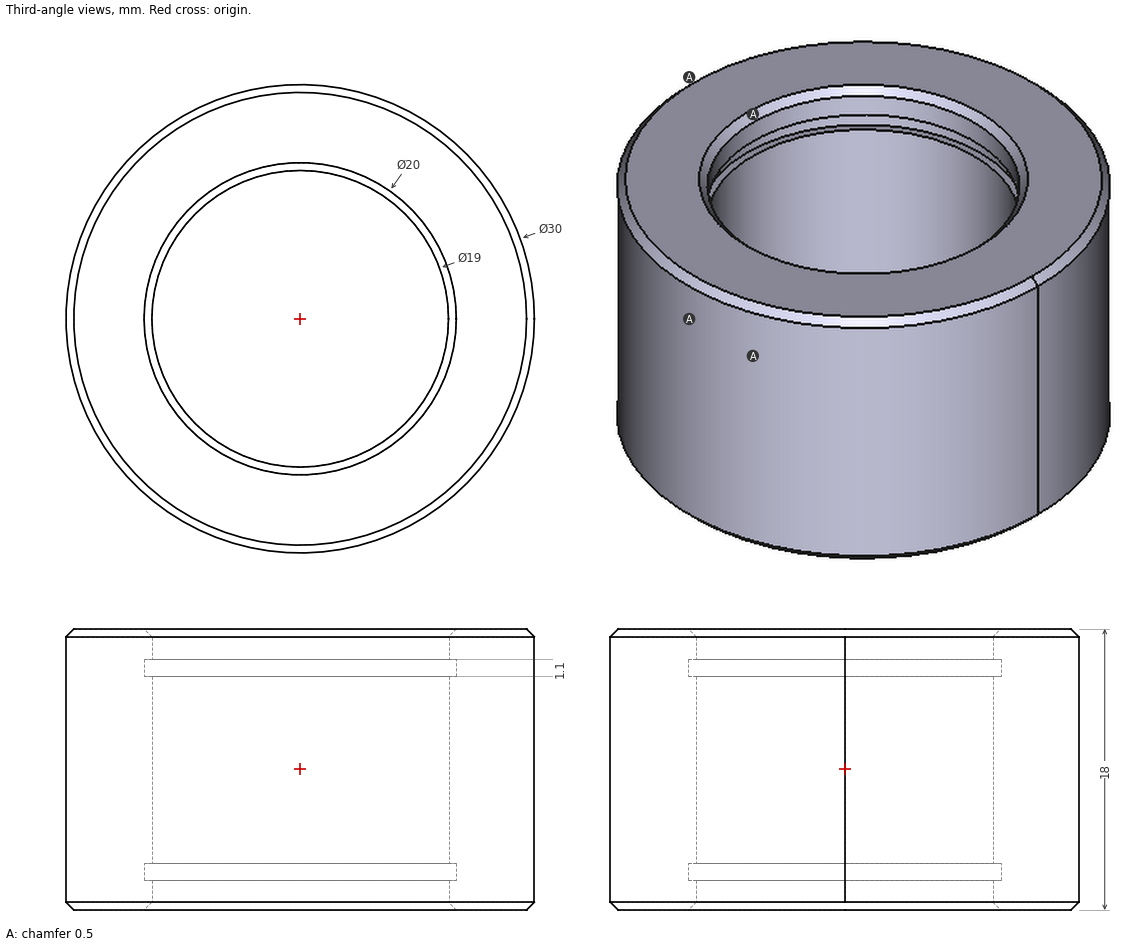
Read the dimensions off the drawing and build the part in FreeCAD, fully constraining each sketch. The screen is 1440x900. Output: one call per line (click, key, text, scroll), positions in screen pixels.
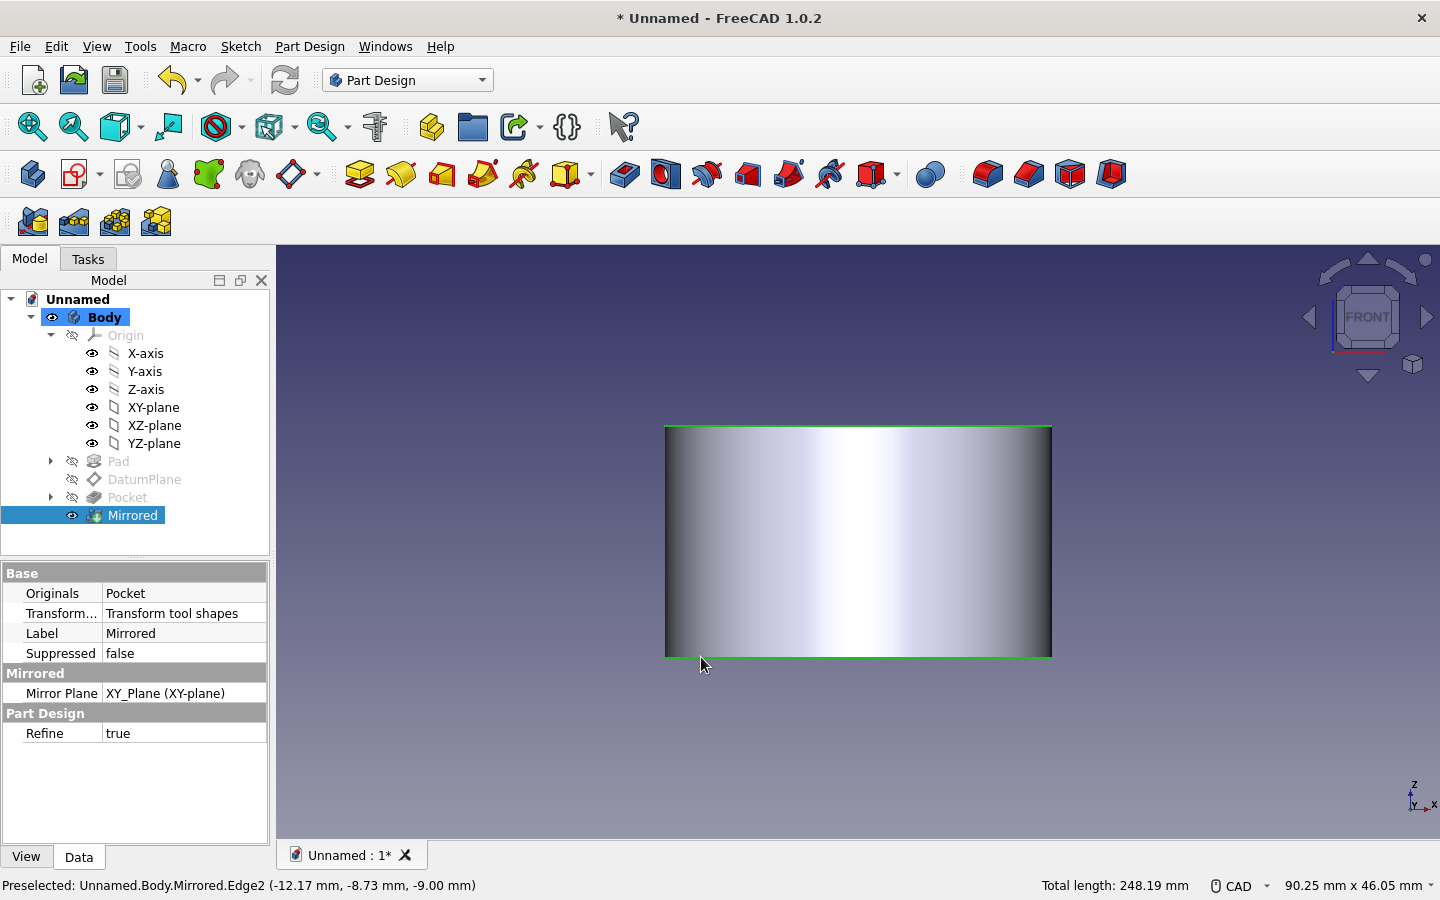
key(3)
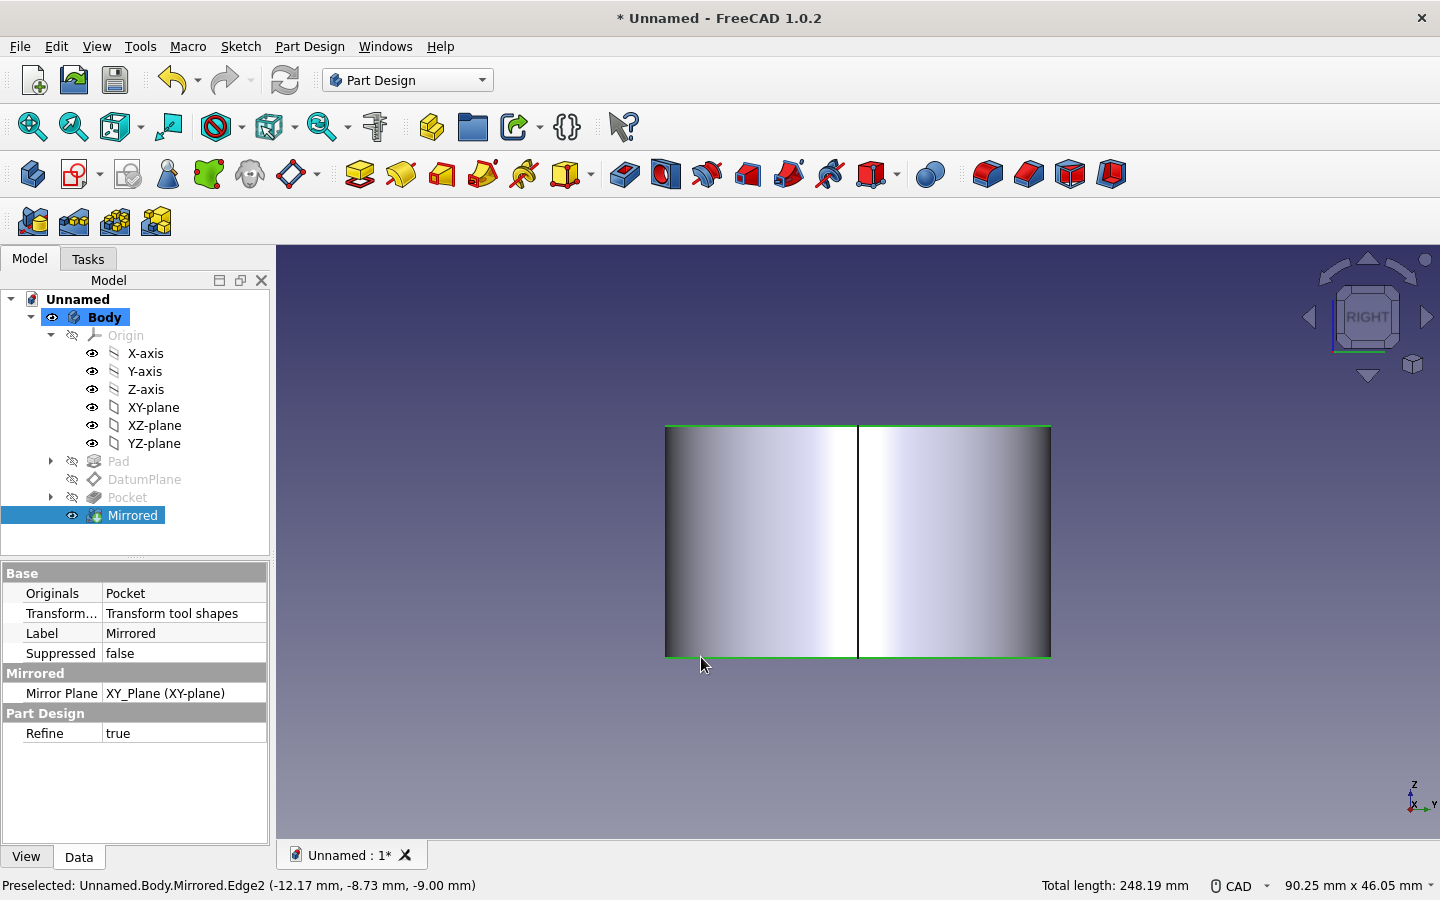
key(v)
key(f)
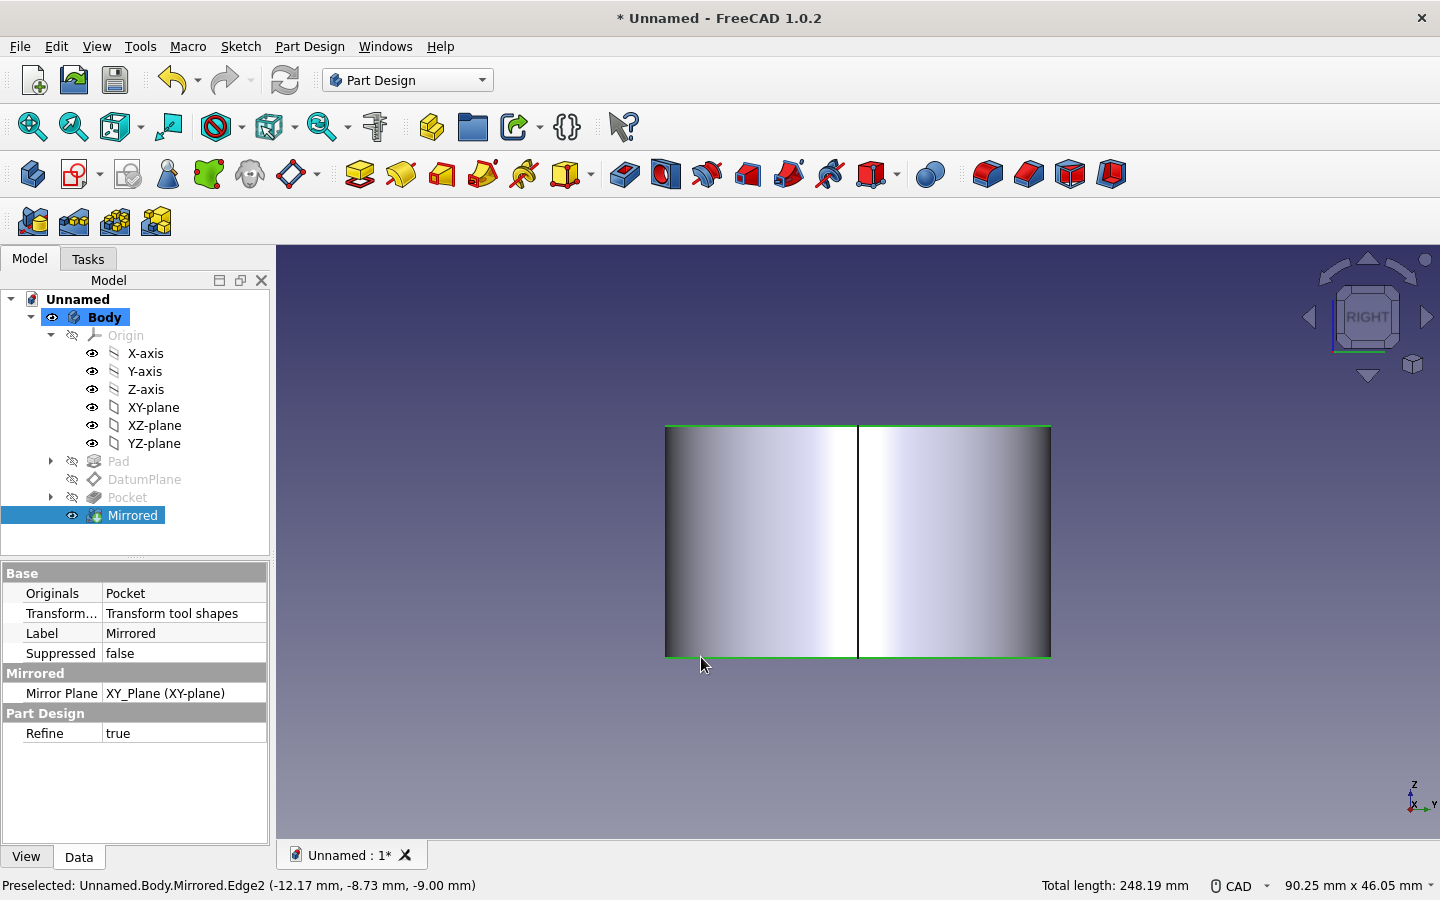
key(5)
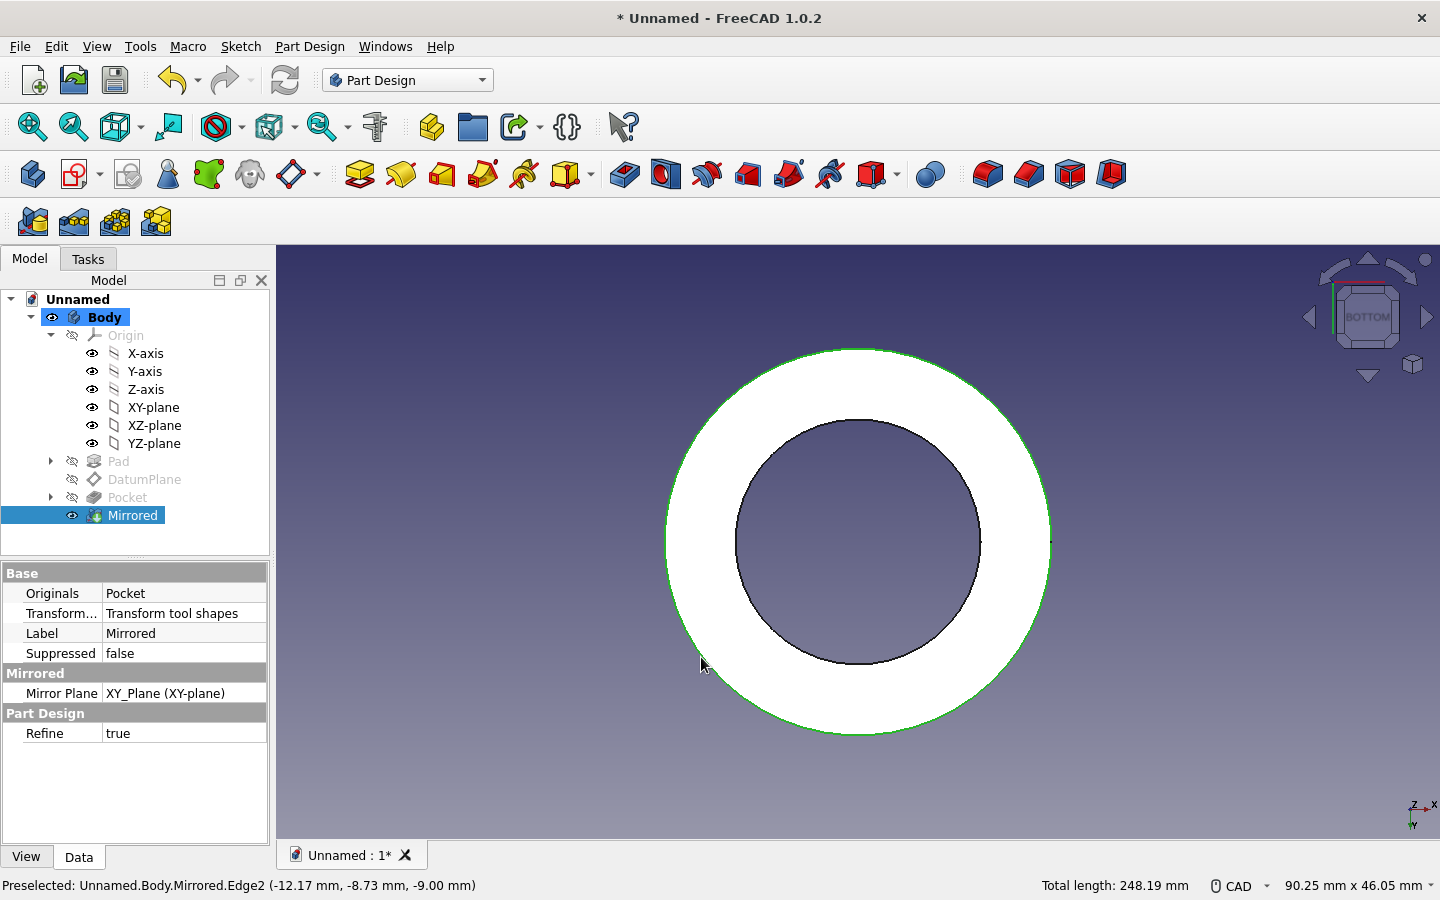
click(735, 541, ctrl)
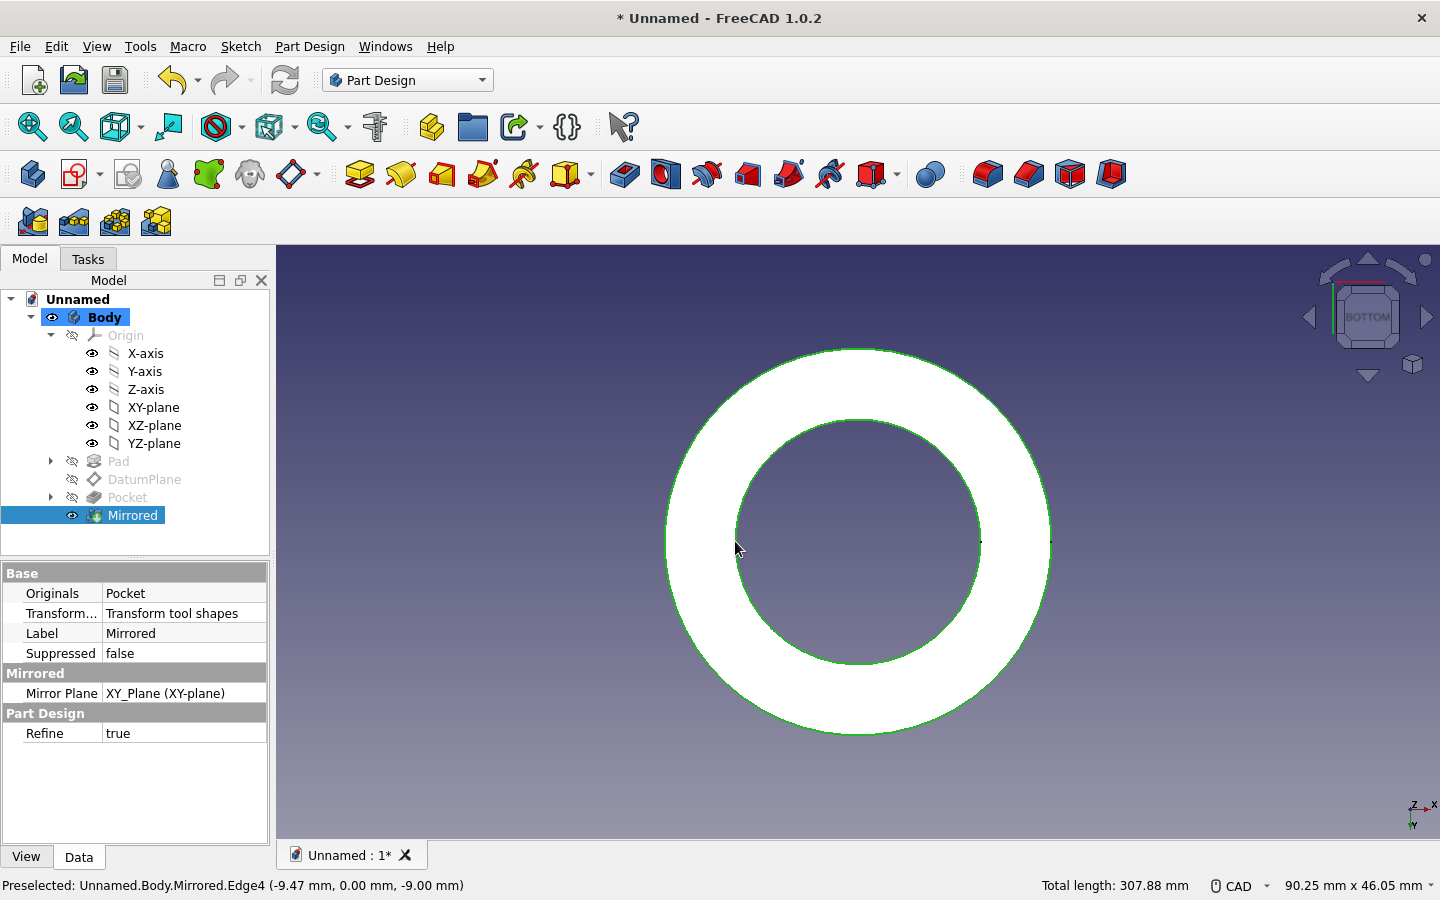
click(1029, 174)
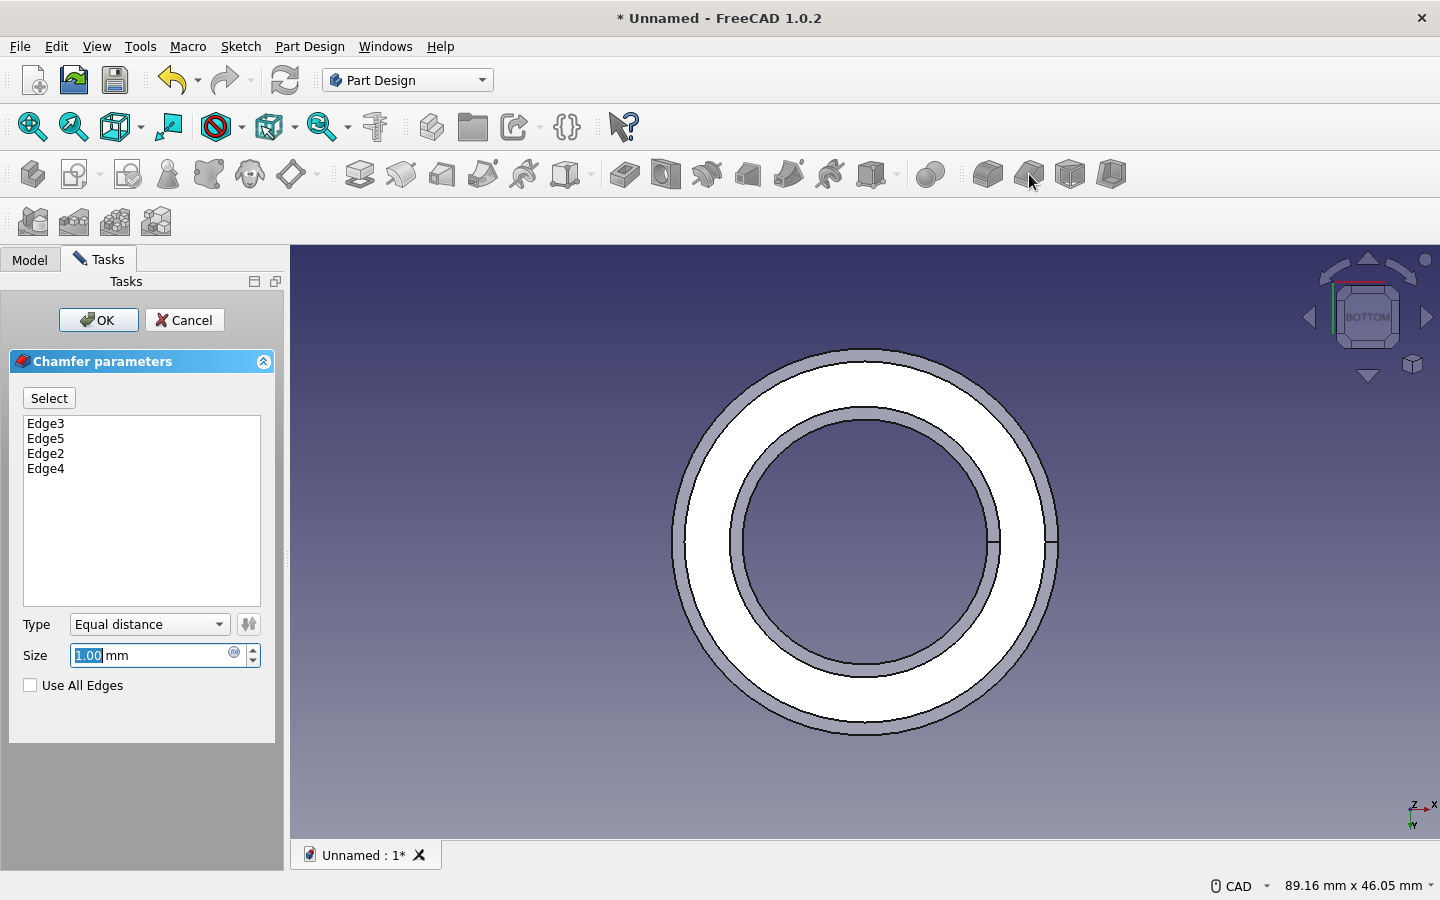
text(0.5)
key(Tab)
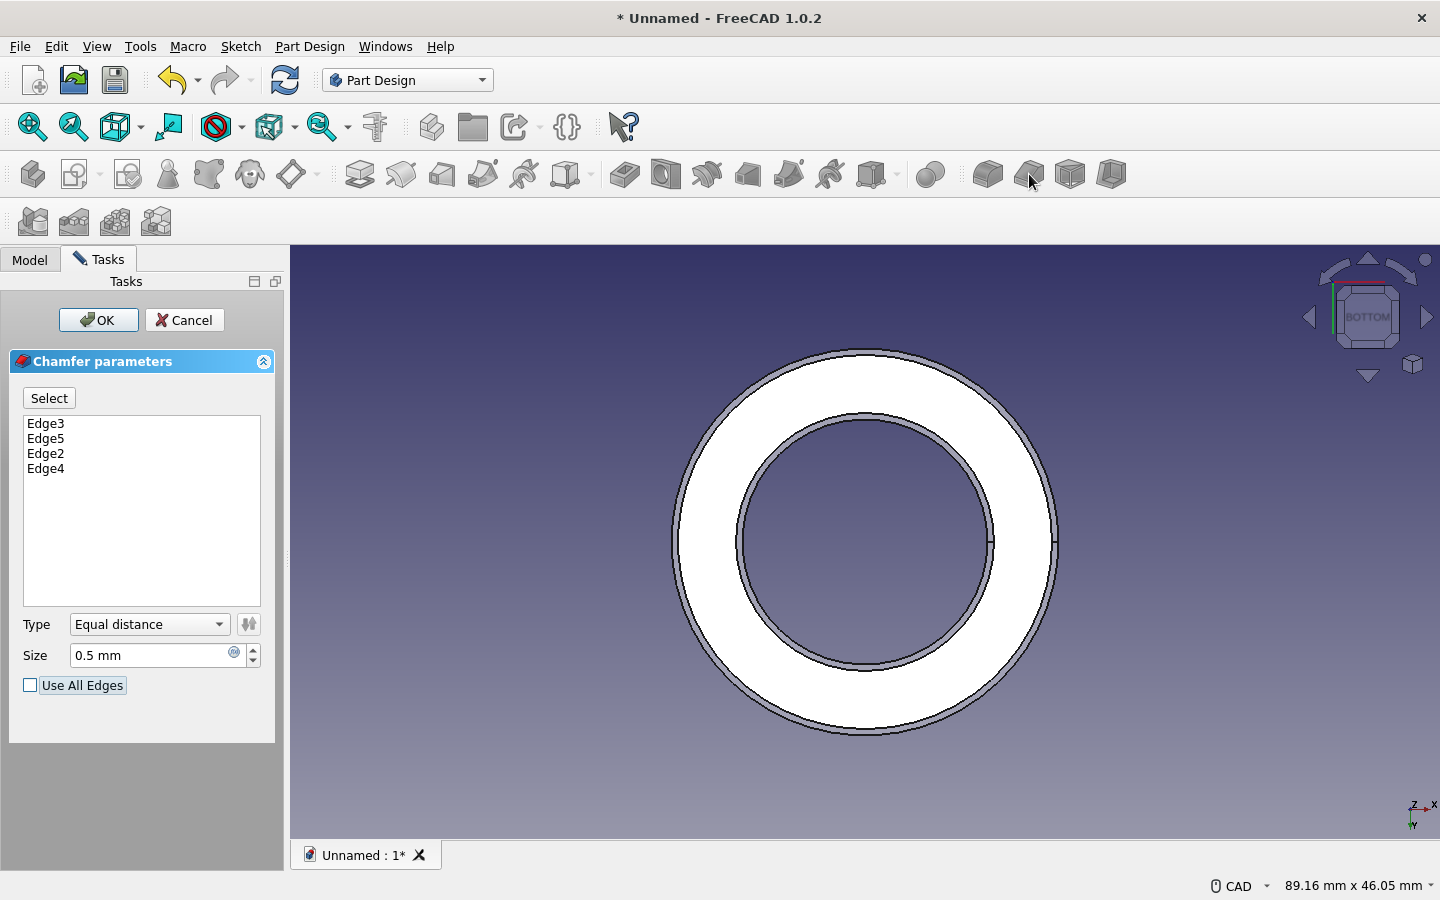
click(99, 320)